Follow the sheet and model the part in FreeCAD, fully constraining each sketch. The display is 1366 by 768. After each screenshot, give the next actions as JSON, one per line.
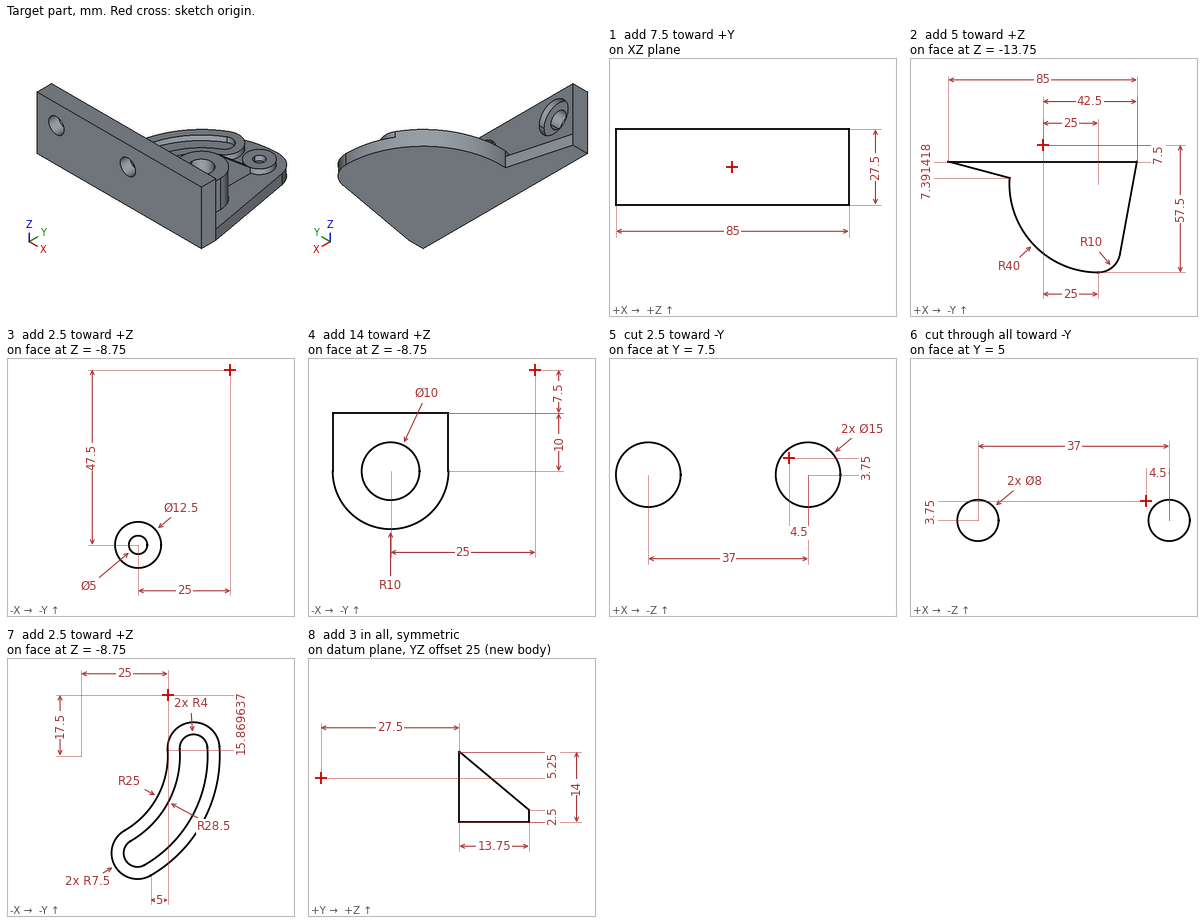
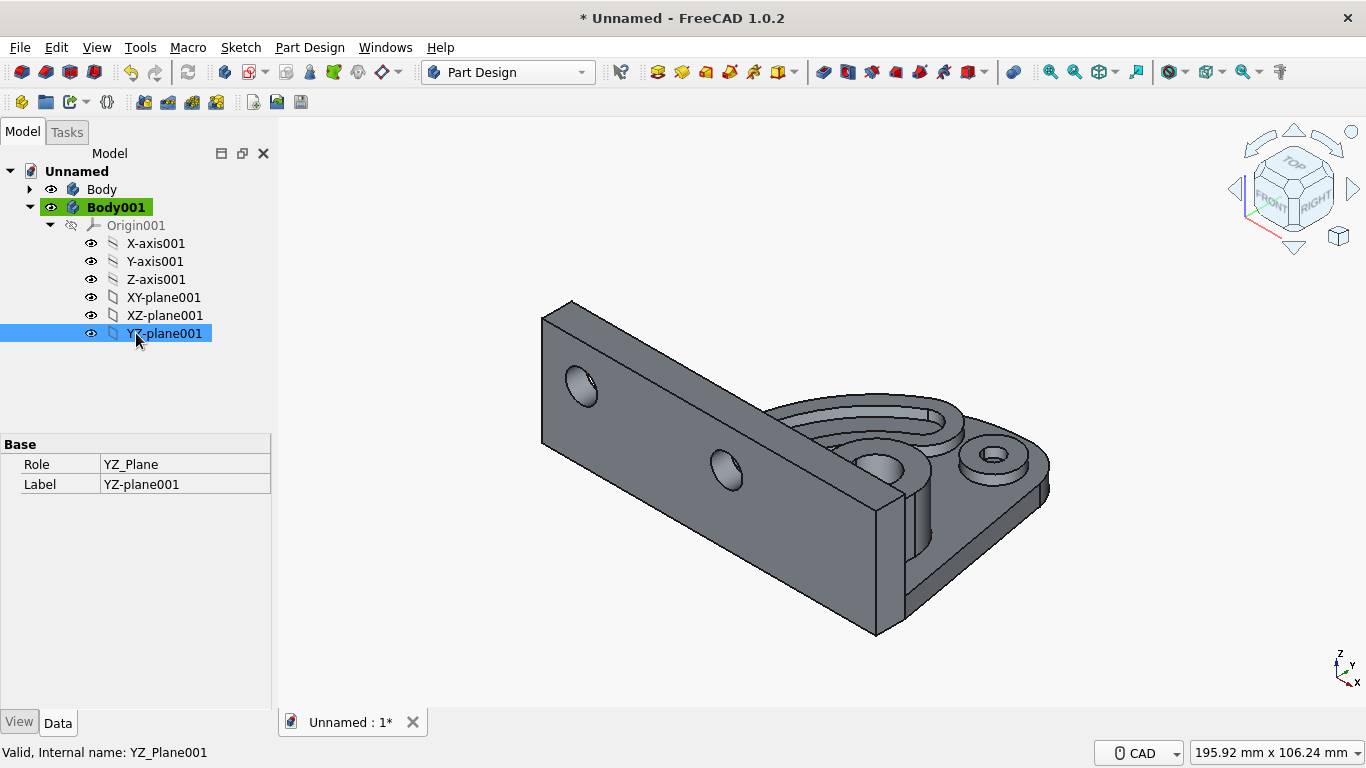
{"action": "left_click", "coordinate": [382, 72]}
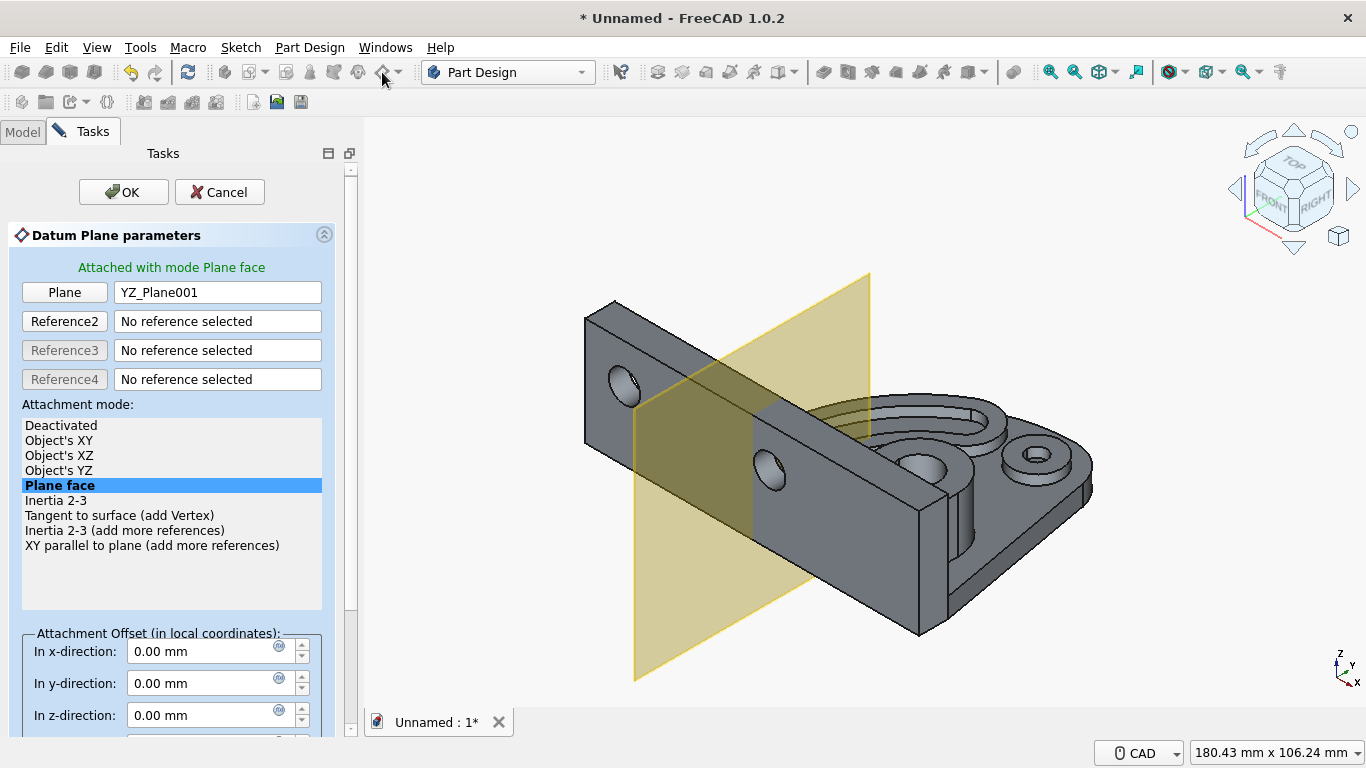
{"action": "triple_click", "coordinate": [210, 715]}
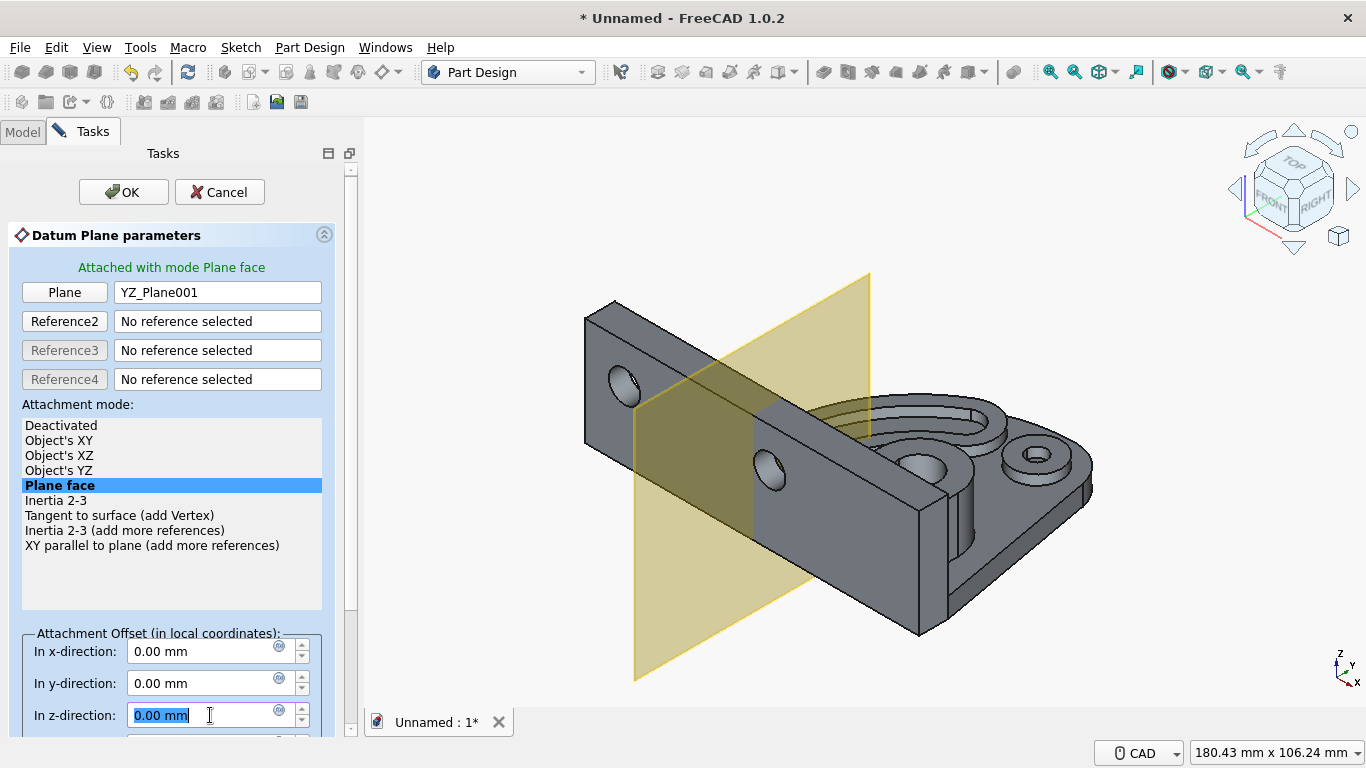
{"action": "type", "text": "25"}
{"action": "key", "text": "Tab"}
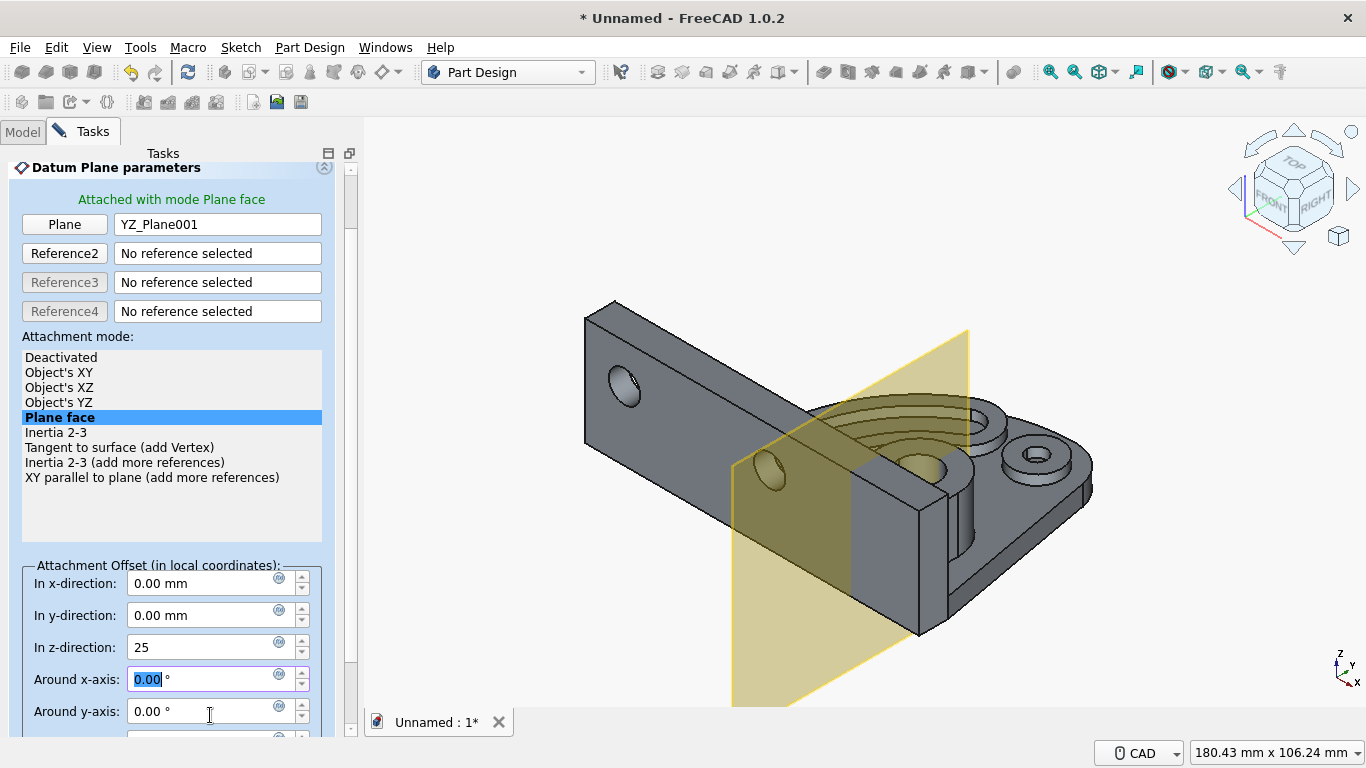
{"action": "scroll", "coordinate": [351, 450], "scroll_direction": "up", "scroll_amount": 2}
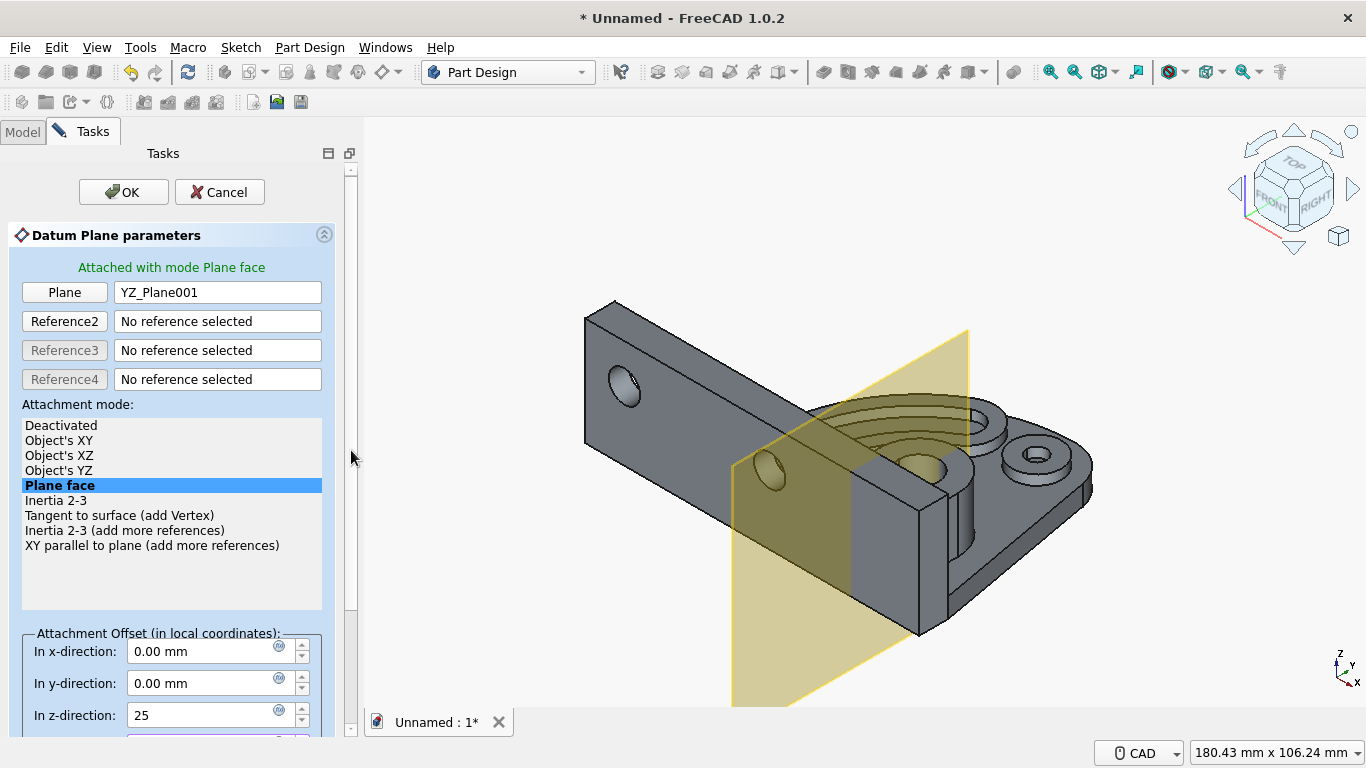
{"action": "left_click", "coordinate": [124, 192]}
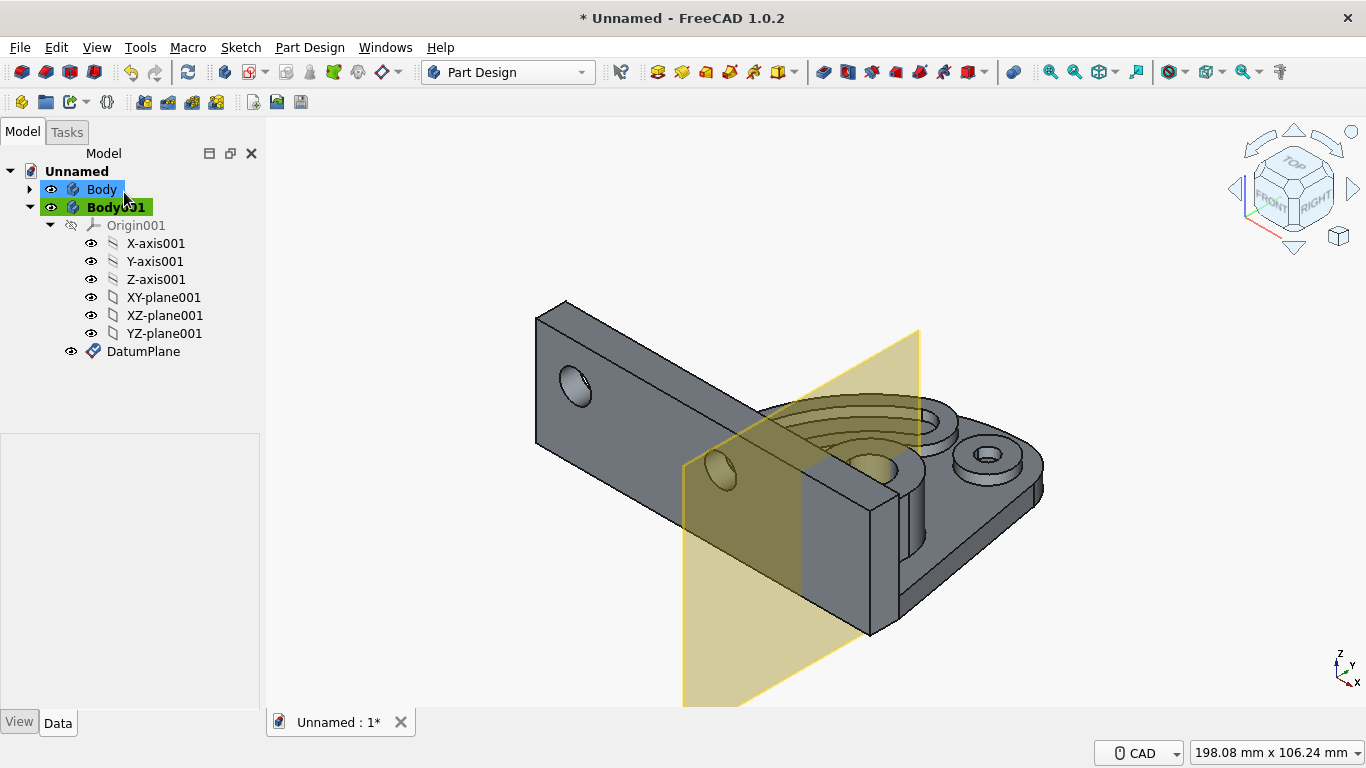
{"action": "left_click", "coordinate": [116, 351]}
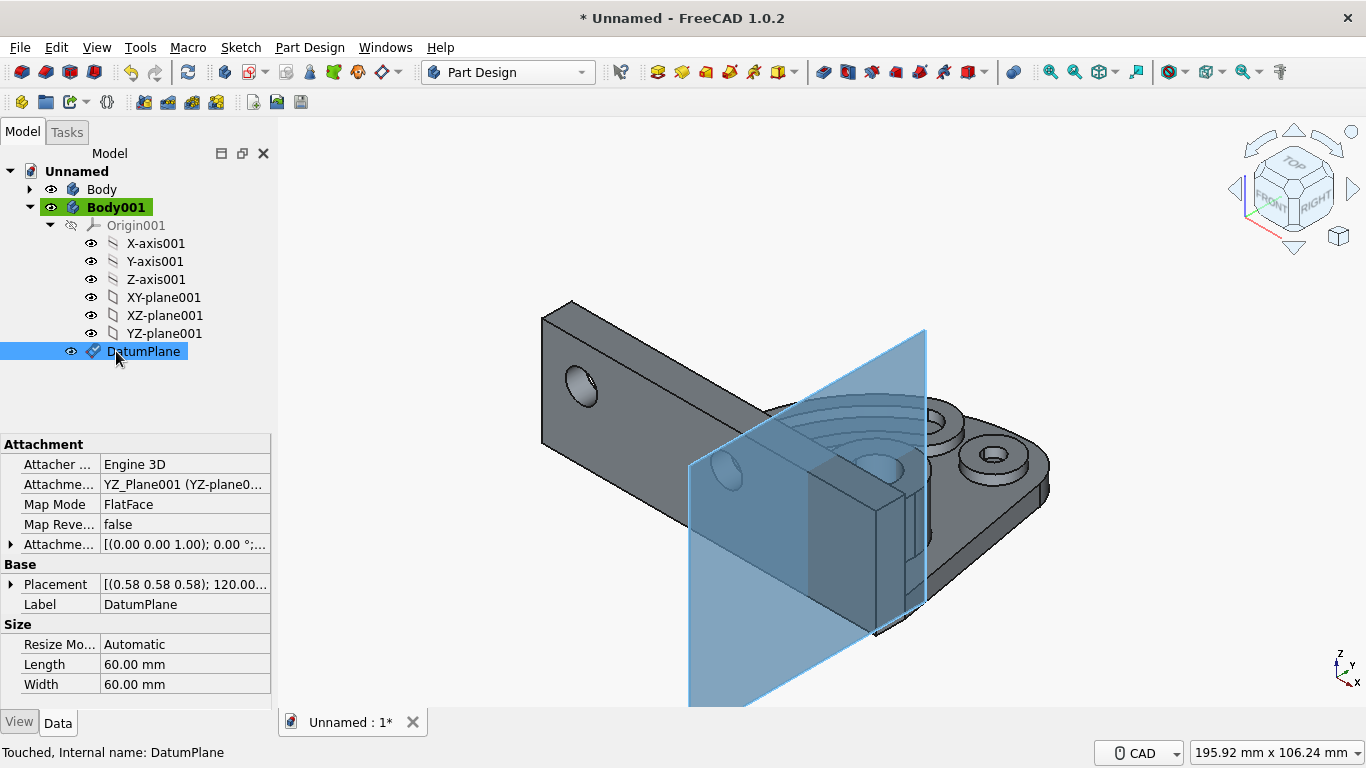
{"action": "left_click", "coordinate": [250, 72]}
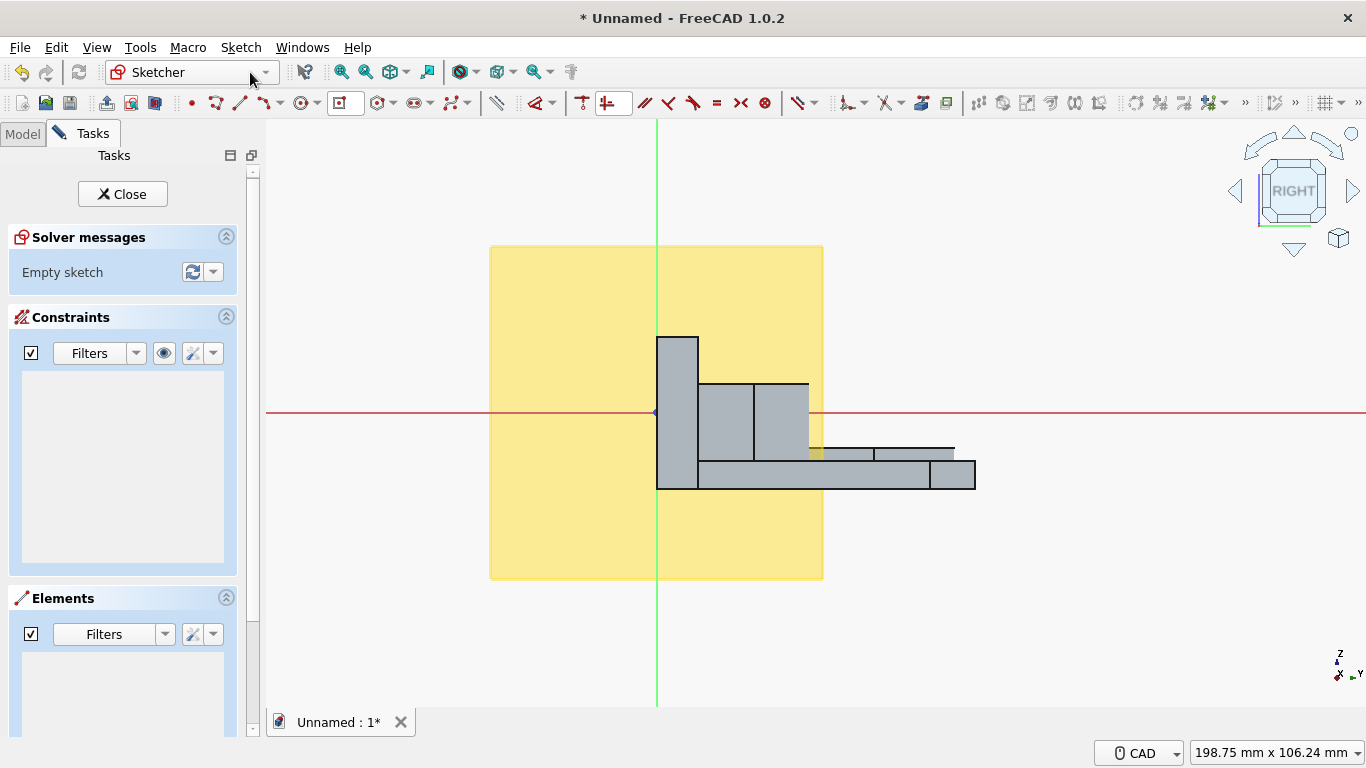
{"action": "scroll", "coordinate": [872, 425], "scroll_direction": "up", "scroll_amount": 8}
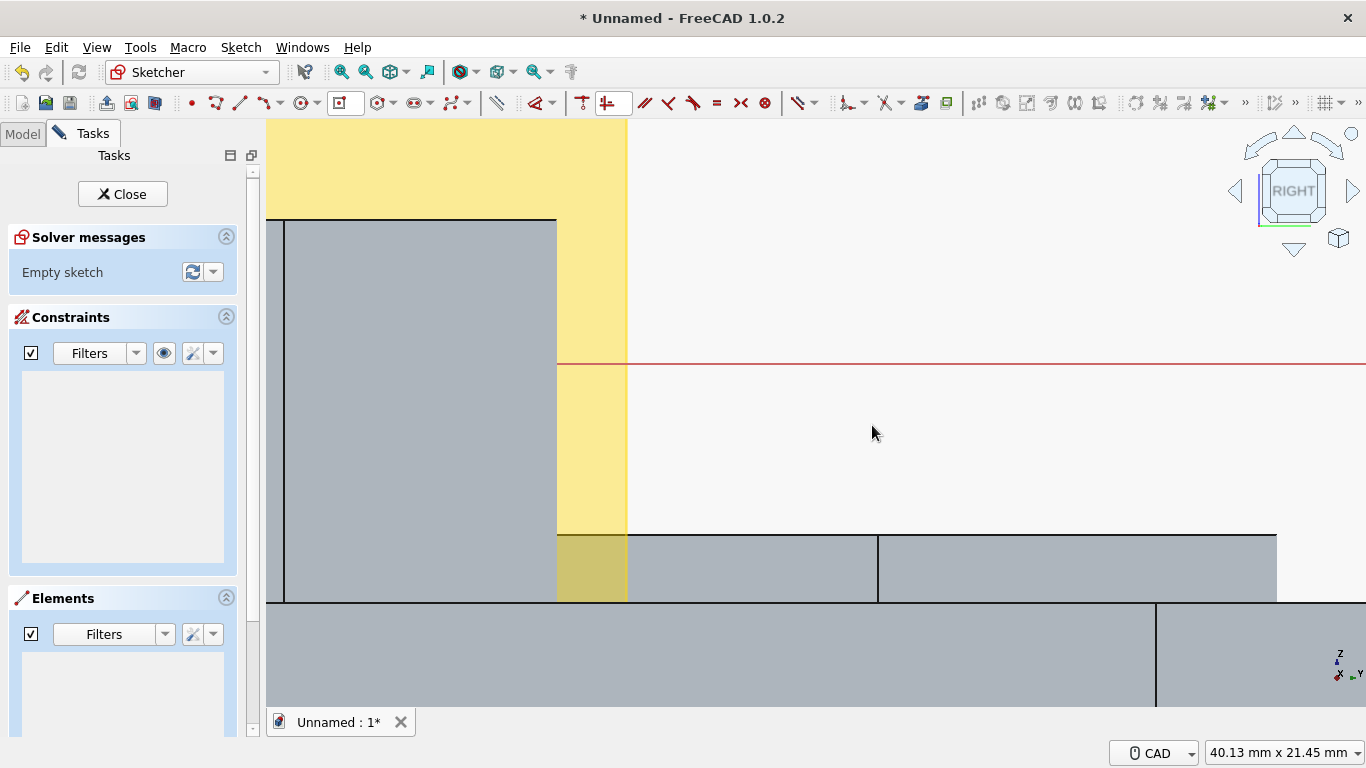
{"action": "left_click", "coordinate": [216, 104]}